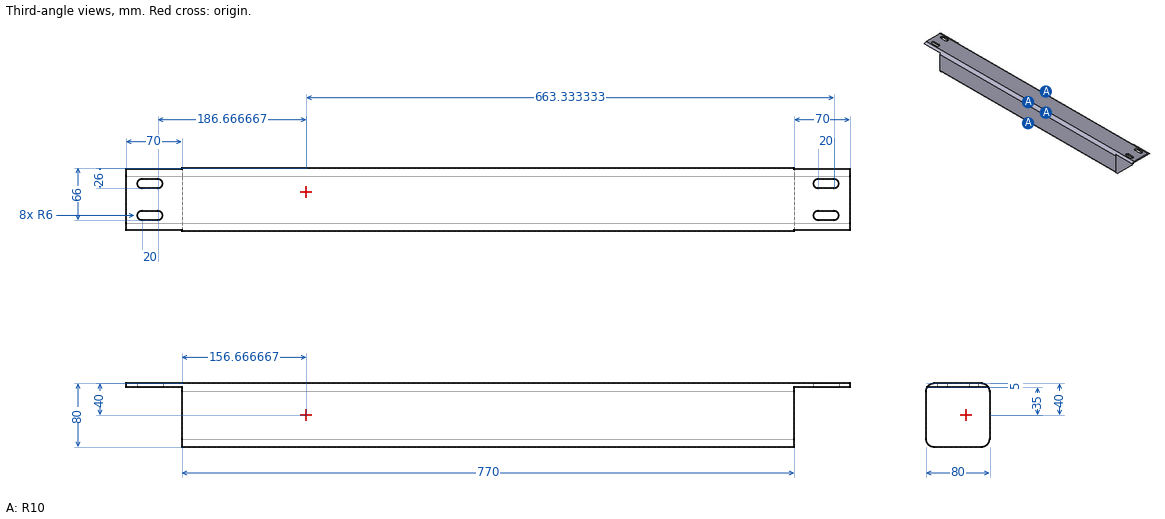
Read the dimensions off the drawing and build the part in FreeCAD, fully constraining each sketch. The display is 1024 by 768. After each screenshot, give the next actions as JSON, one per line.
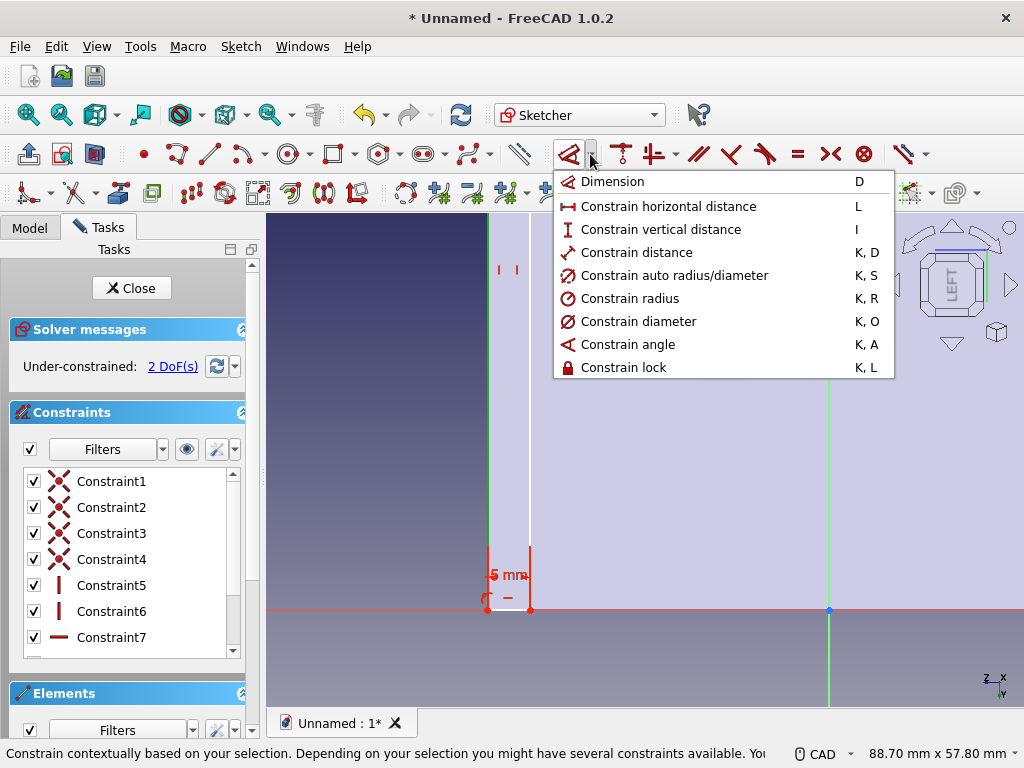
{"action": "left_click", "coordinate": [724, 230]}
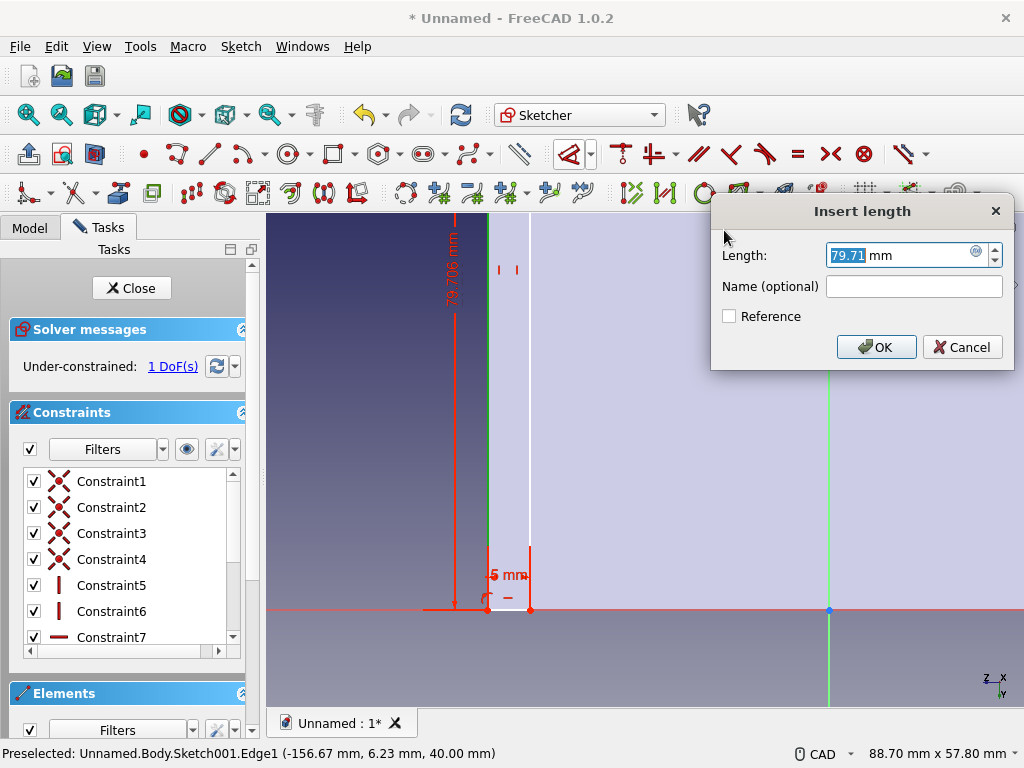
{"action": "type", "text": "80"}
{"action": "key", "text": "Return"}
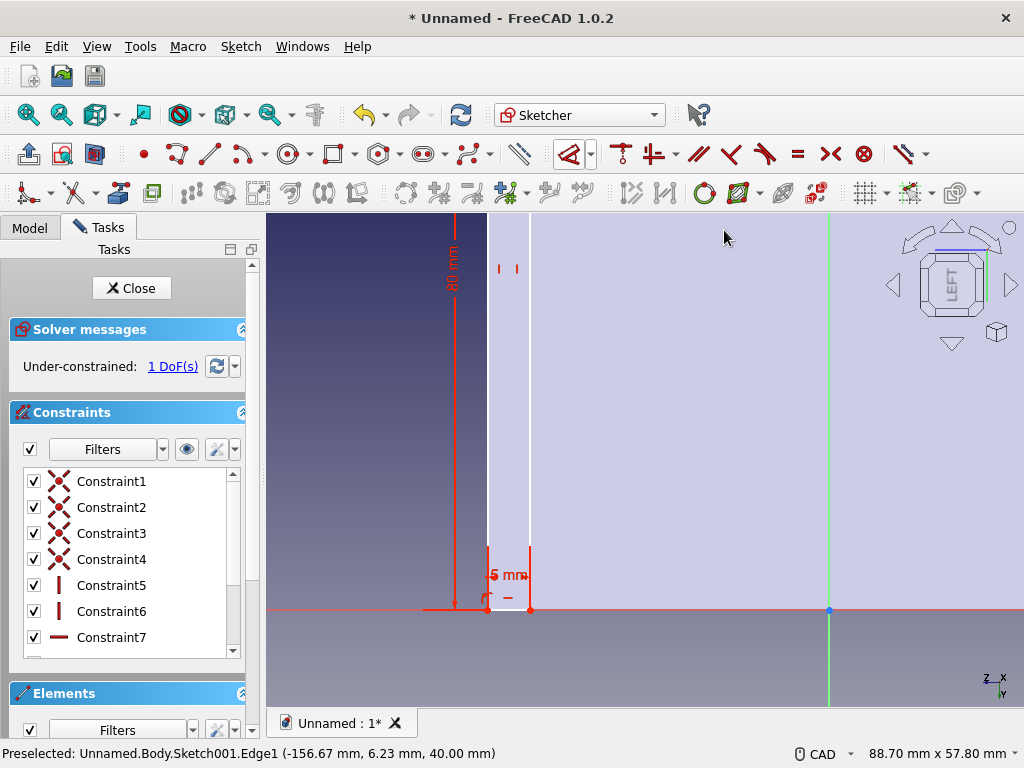
{"action": "scroll", "coordinate": [510, 616], "scroll_direction": "down", "scroll_amount": 4}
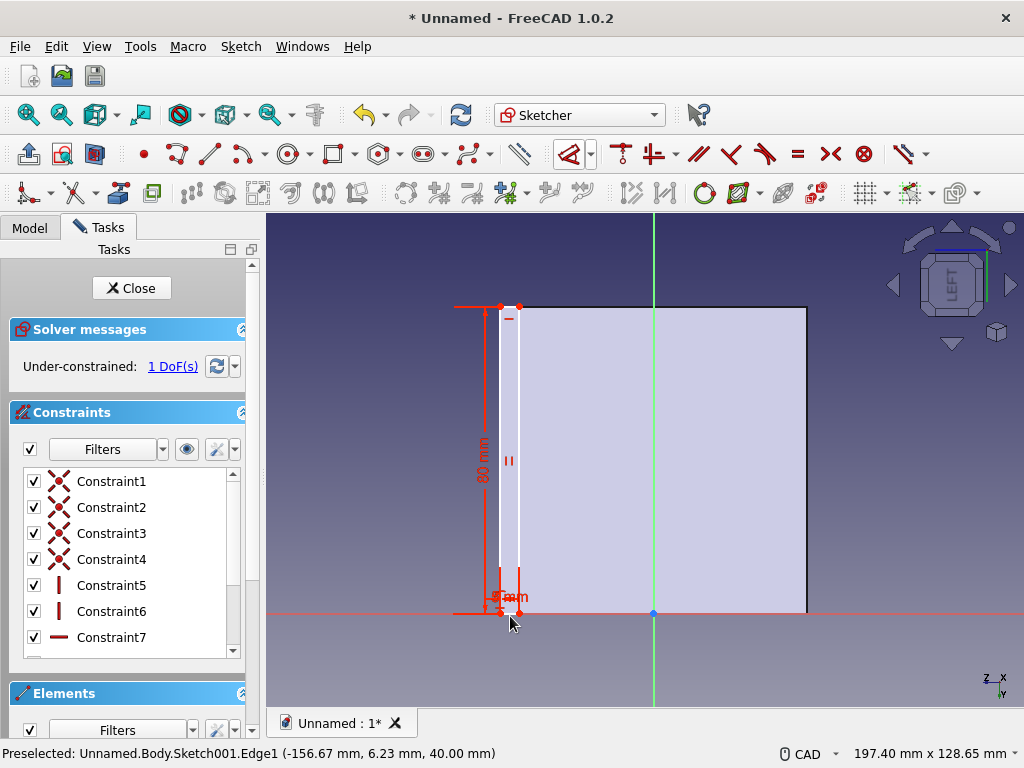
{"action": "left_click", "coordinate": [500, 307]}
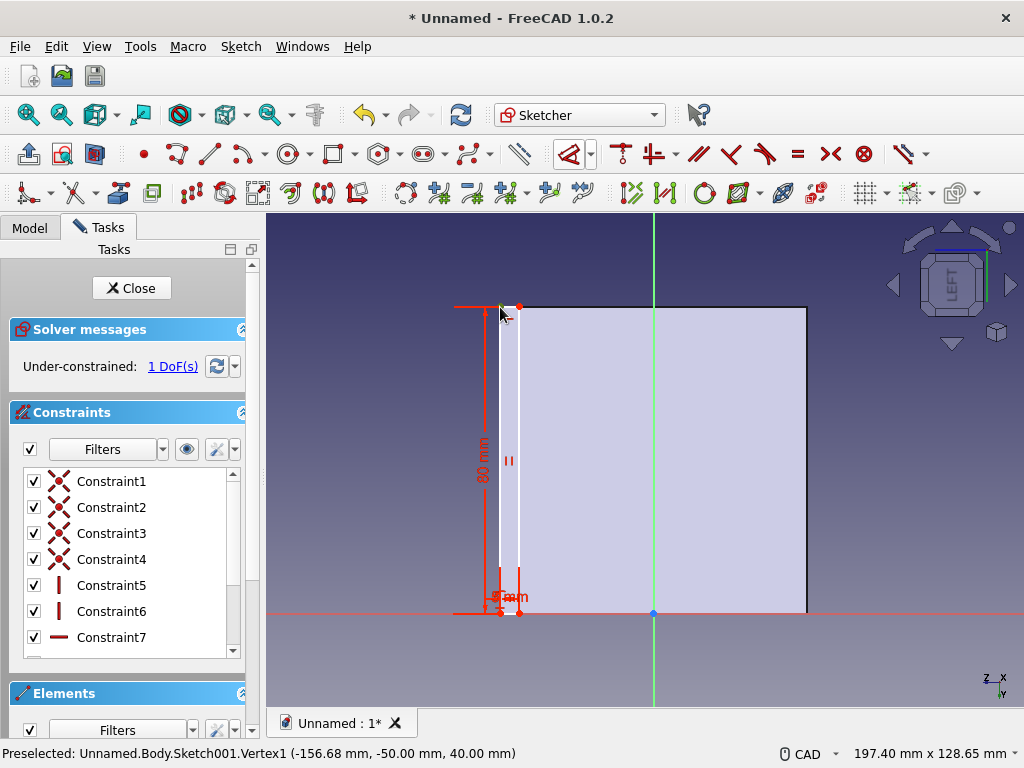
{"action": "key", "text": "l"}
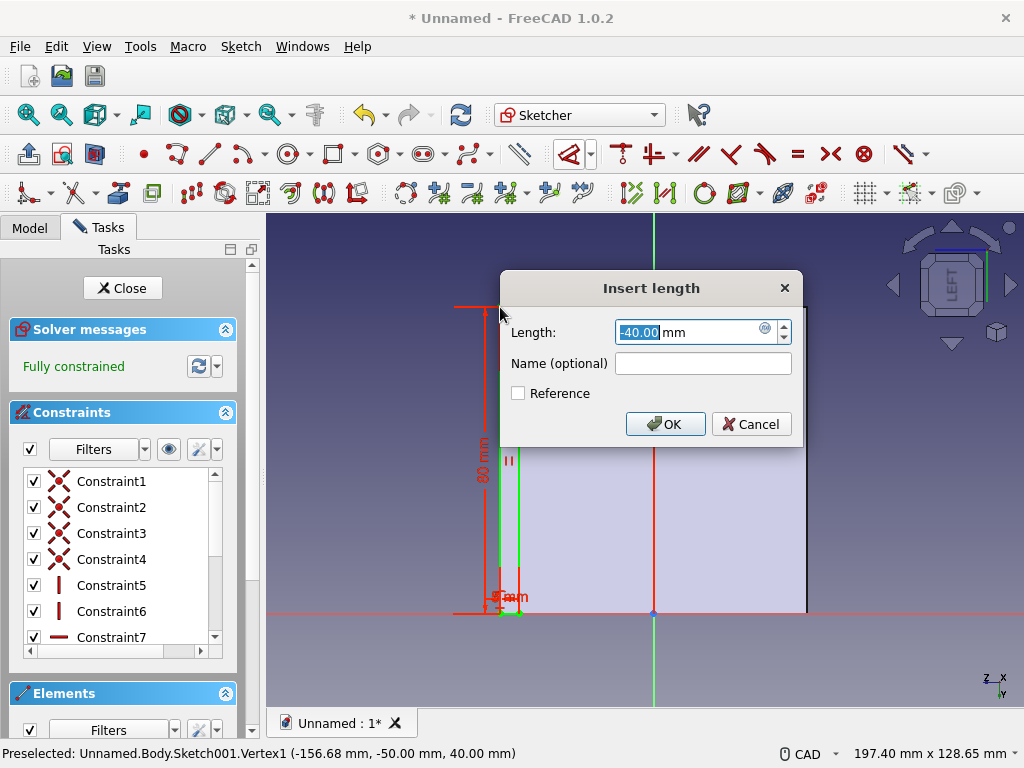
{"action": "type", "text": "-40"}
{"action": "key", "text": "Return"}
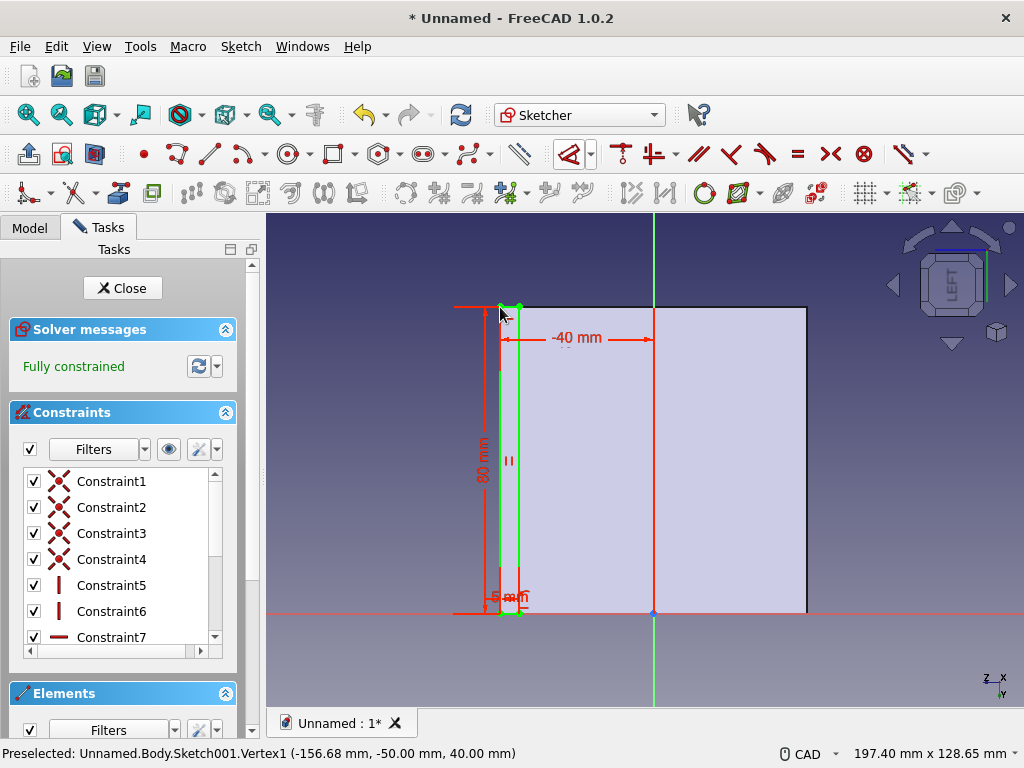
{"action": "left_click", "coordinate": [123, 288]}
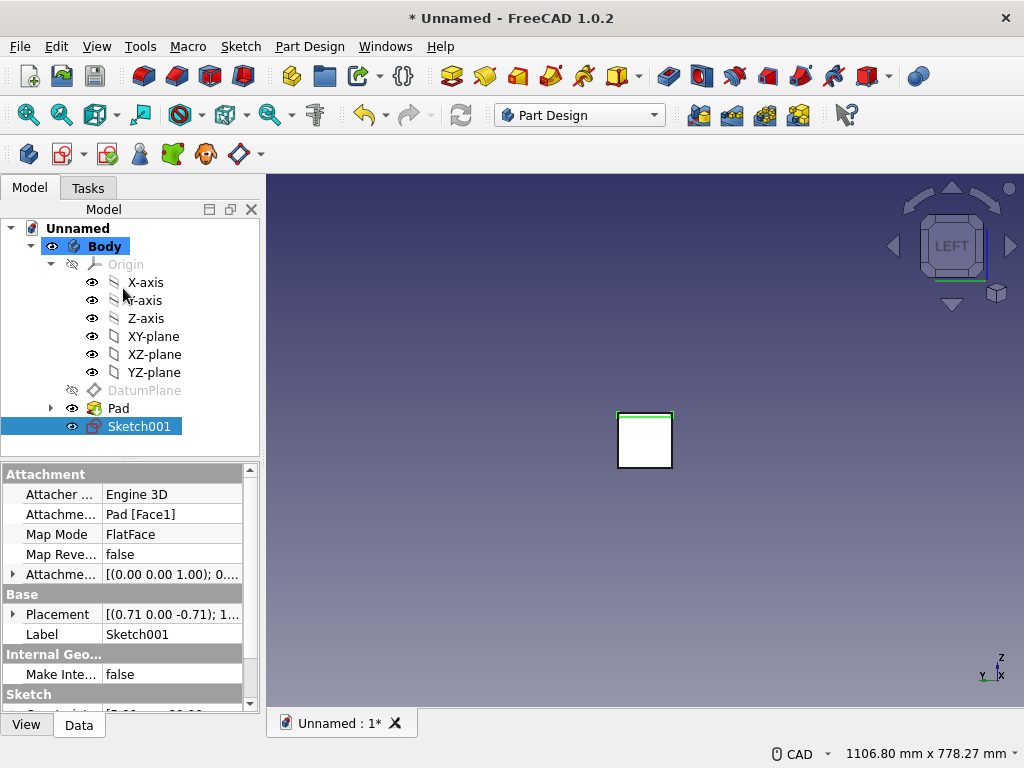
{"action": "left_click", "coordinate": [452, 76]}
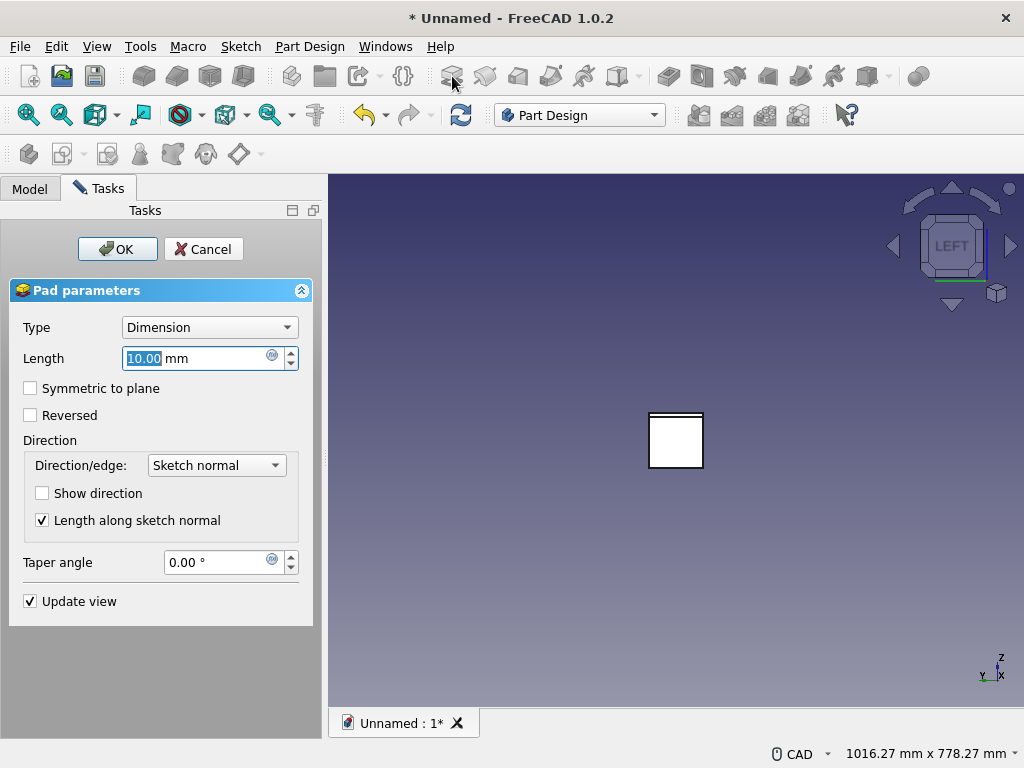
{"action": "type", "text": "70"}
{"action": "key", "text": "Tab"}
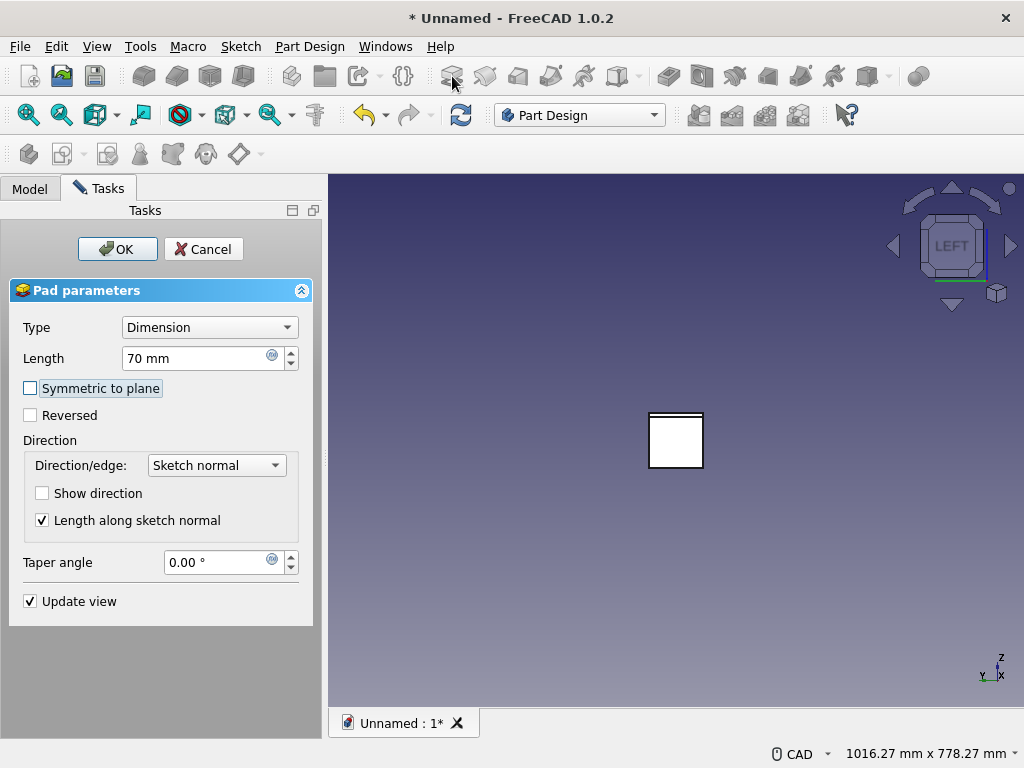
{"action": "left_click", "coordinate": [118, 249]}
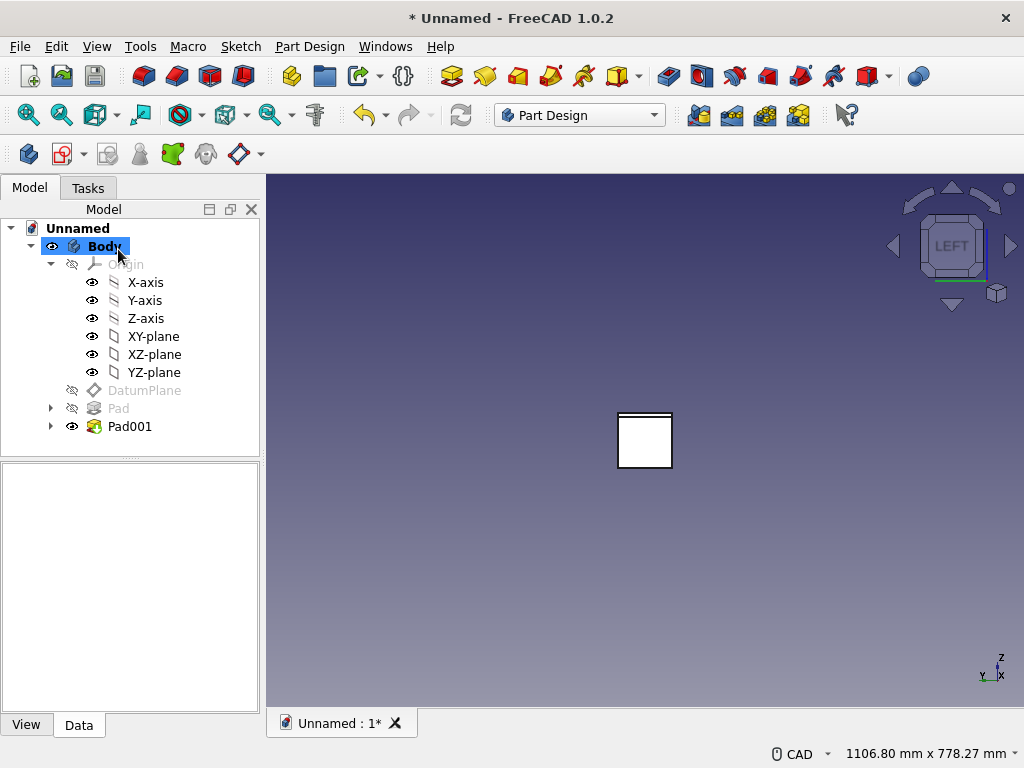
{"action": "left_click", "coordinate": [29, 116]}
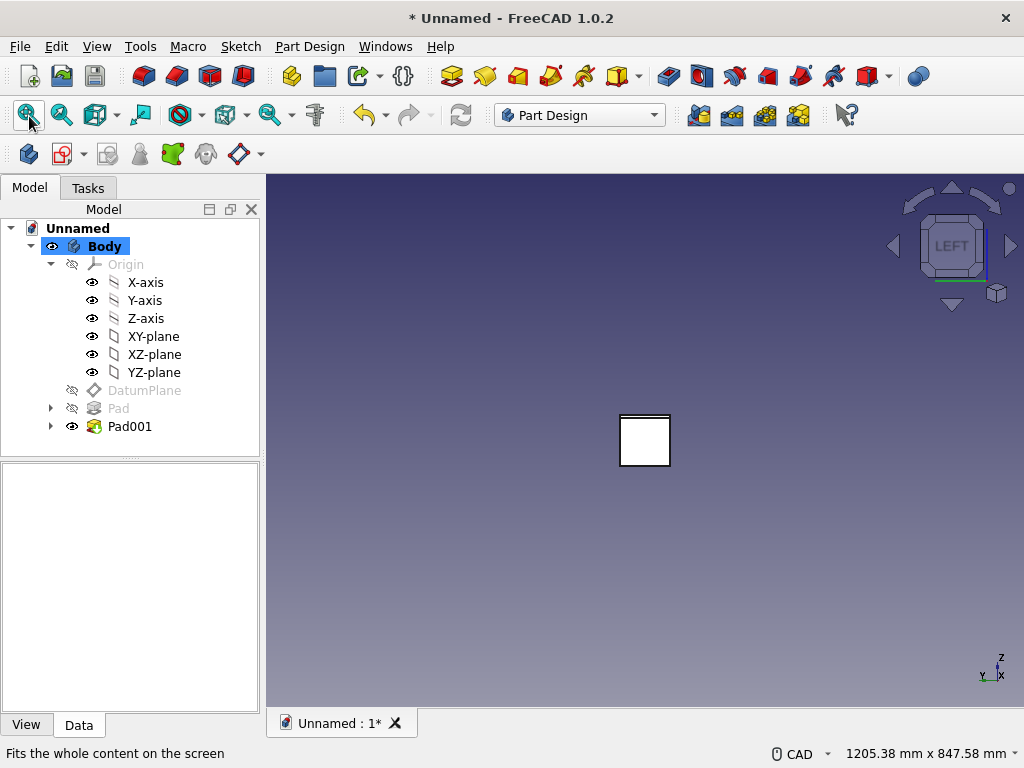
{"action": "key", "text": "0"}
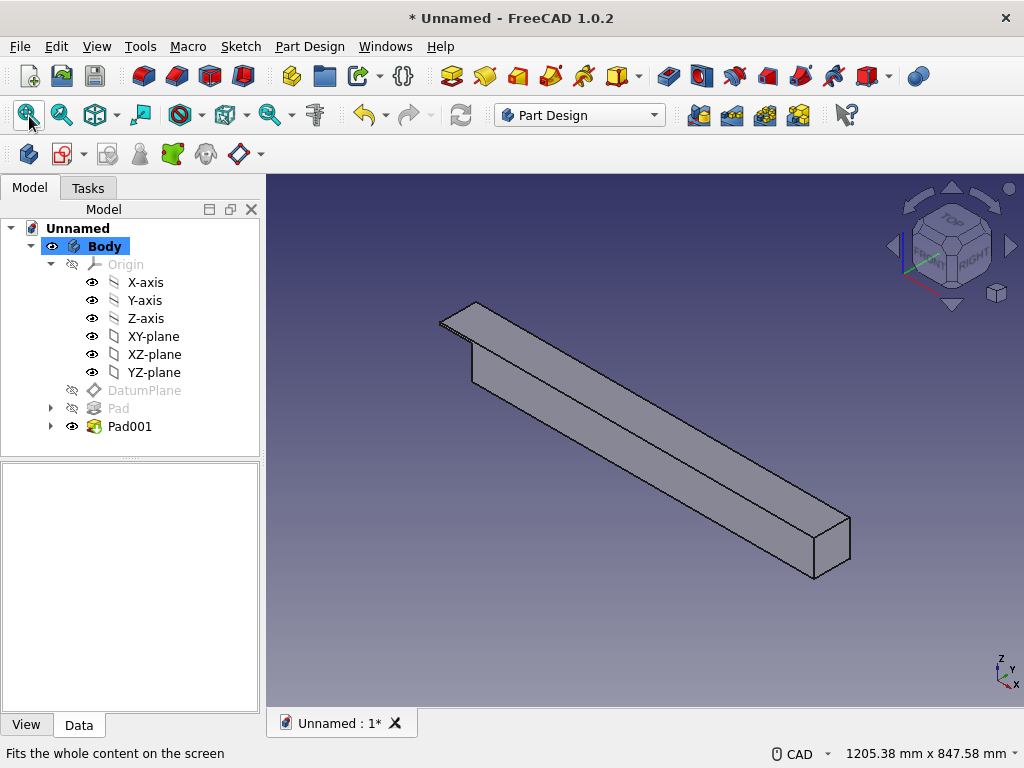
{"action": "left_click", "coordinate": [832, 547]}